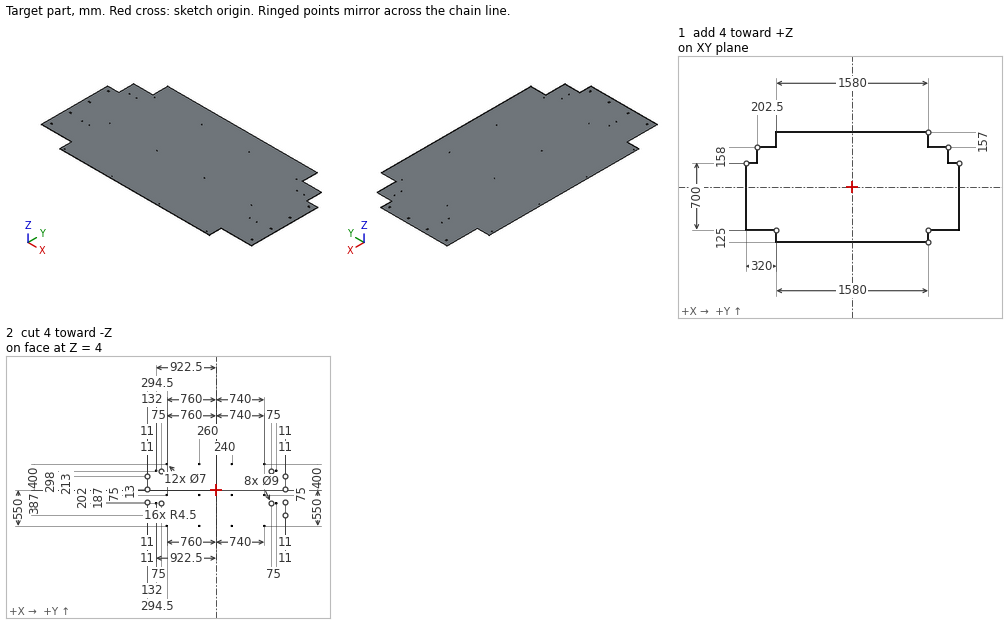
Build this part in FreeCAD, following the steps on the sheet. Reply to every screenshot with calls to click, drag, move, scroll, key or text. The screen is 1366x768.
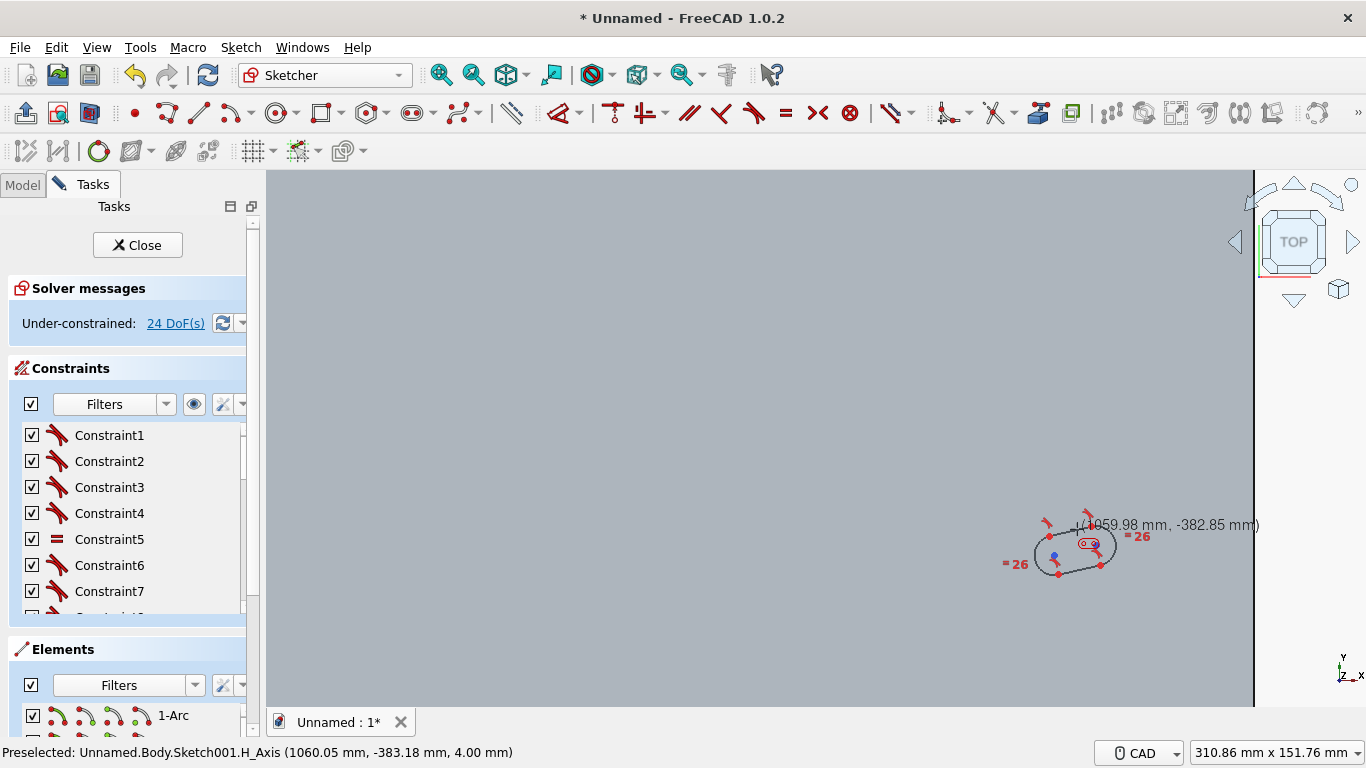
scroll(1089, 538, down, 12)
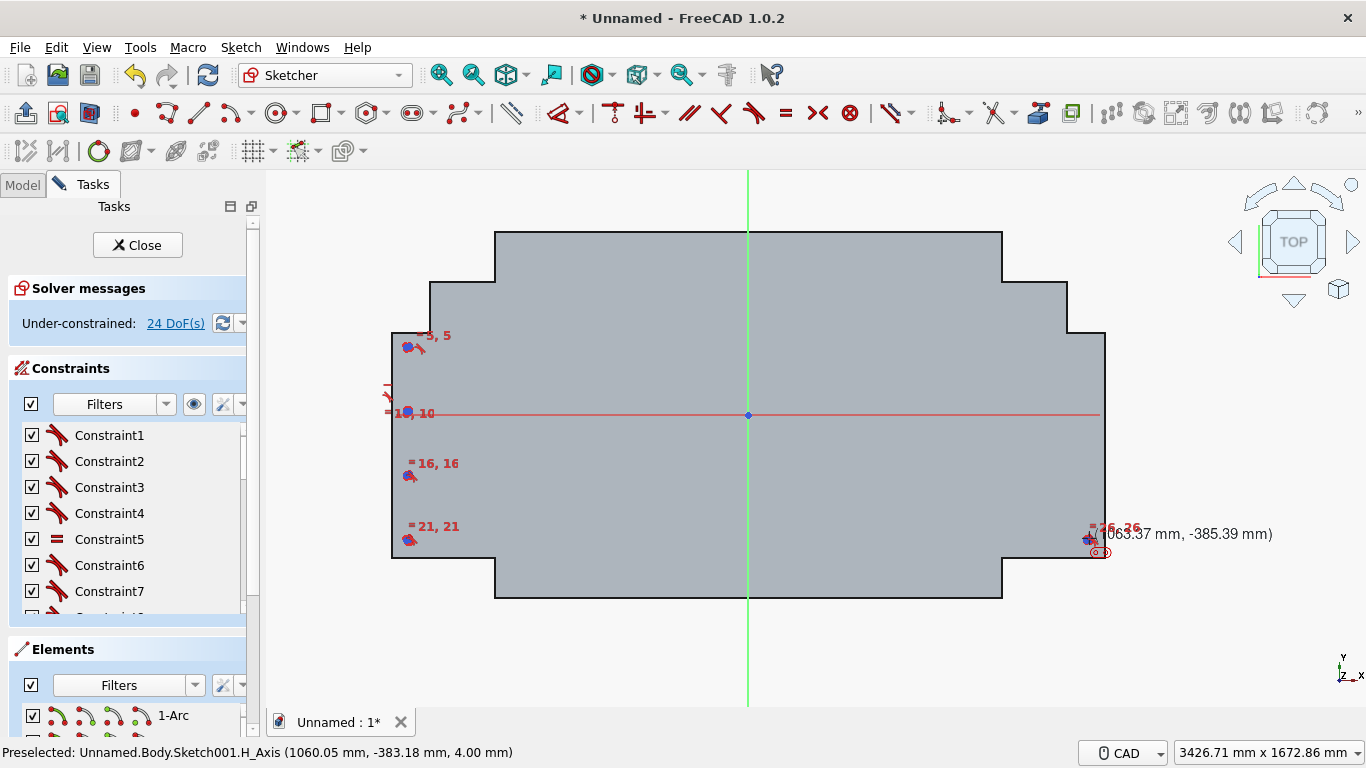
scroll(1087, 475, up, 14)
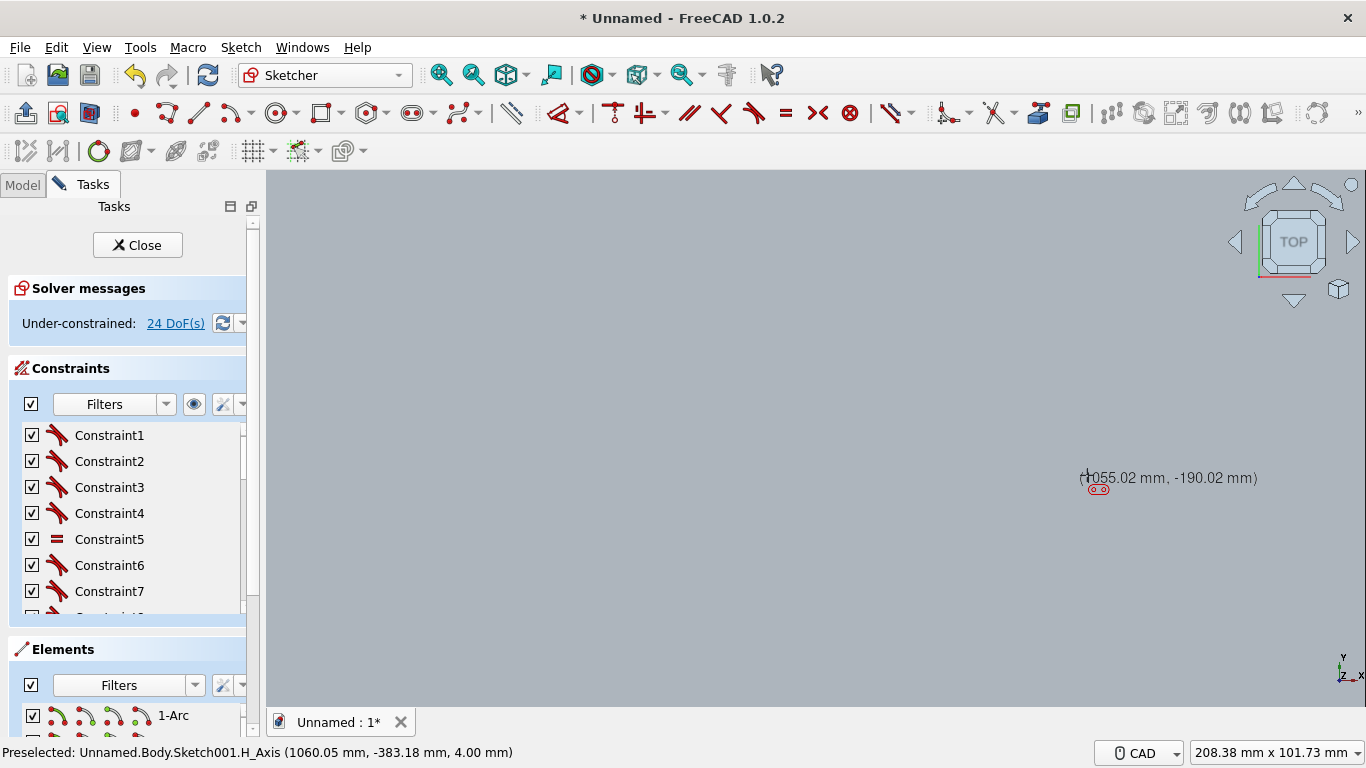
scroll(1087, 475, down, 14)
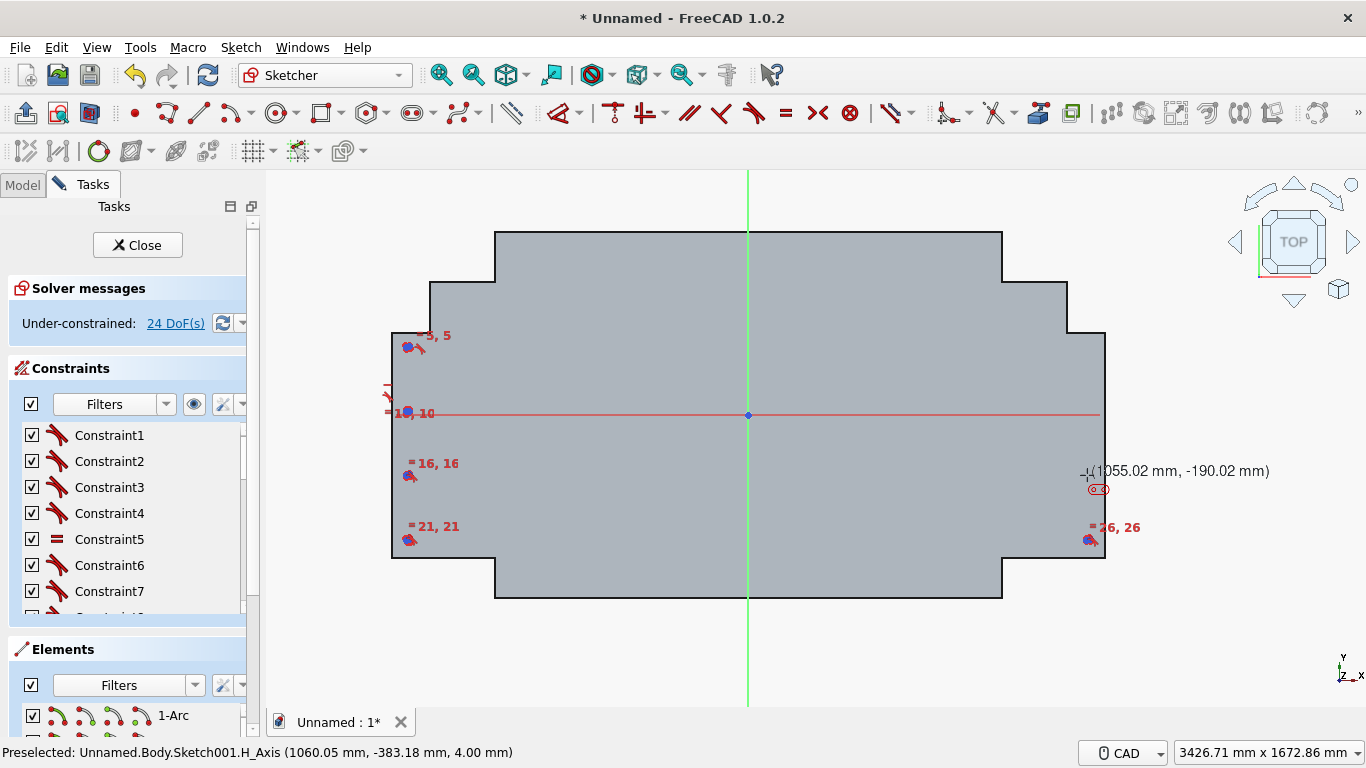
click(1087, 475)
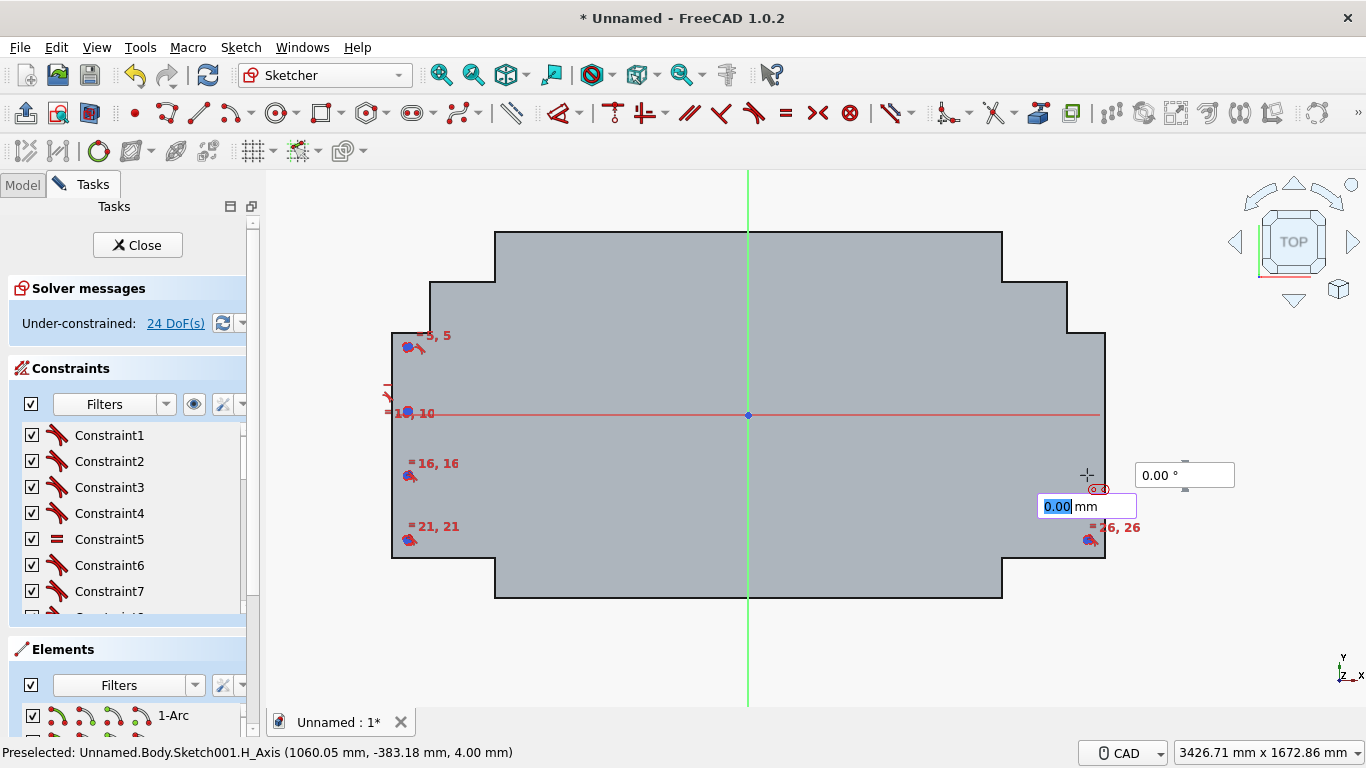
scroll(1090, 475, up, 8)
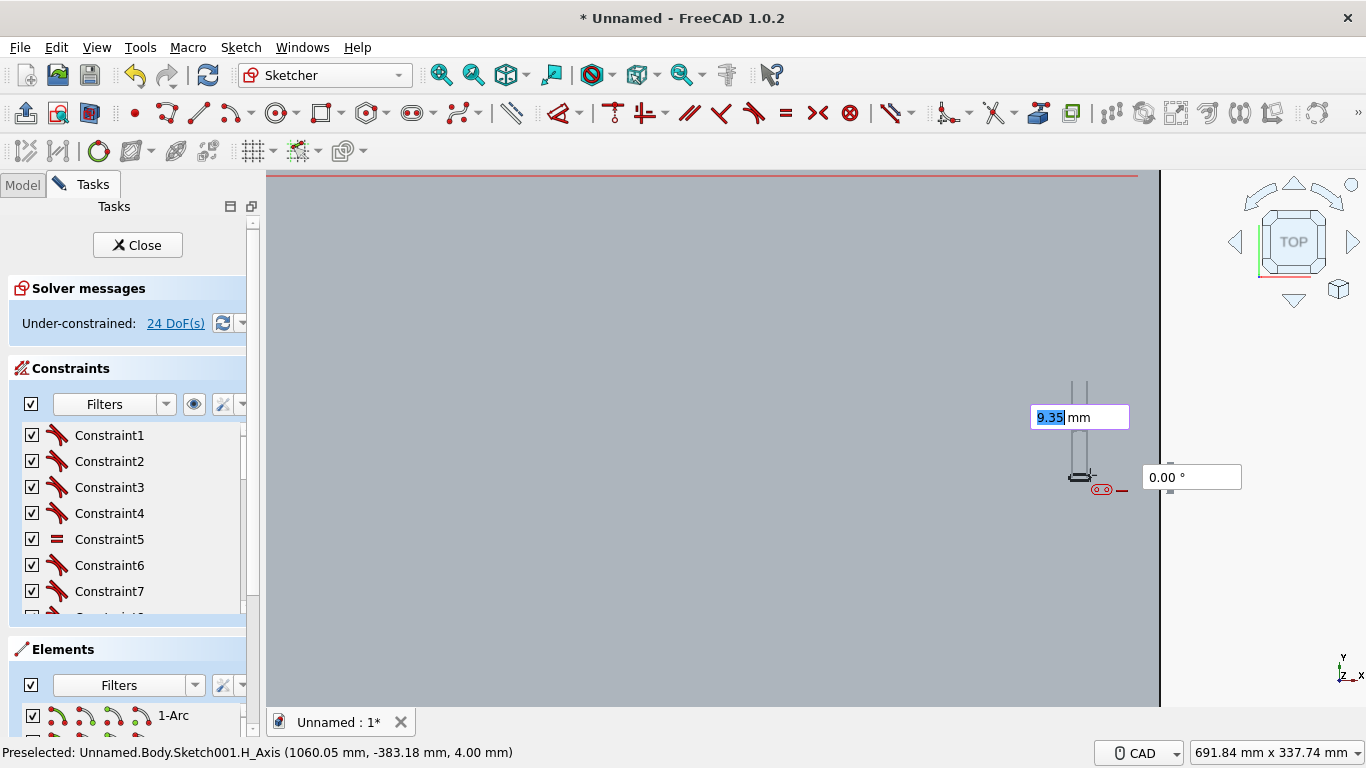
click(1089, 473)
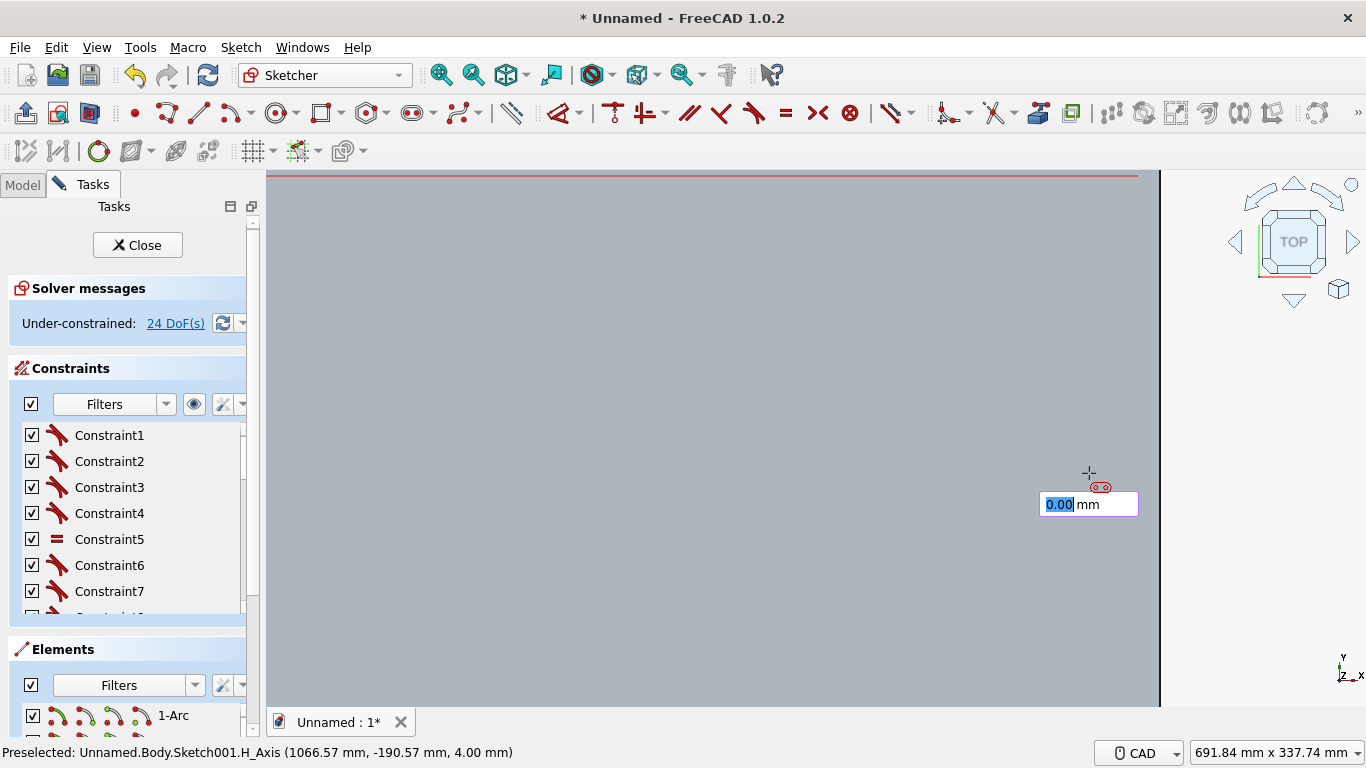
scroll(1080, 466, up, 4)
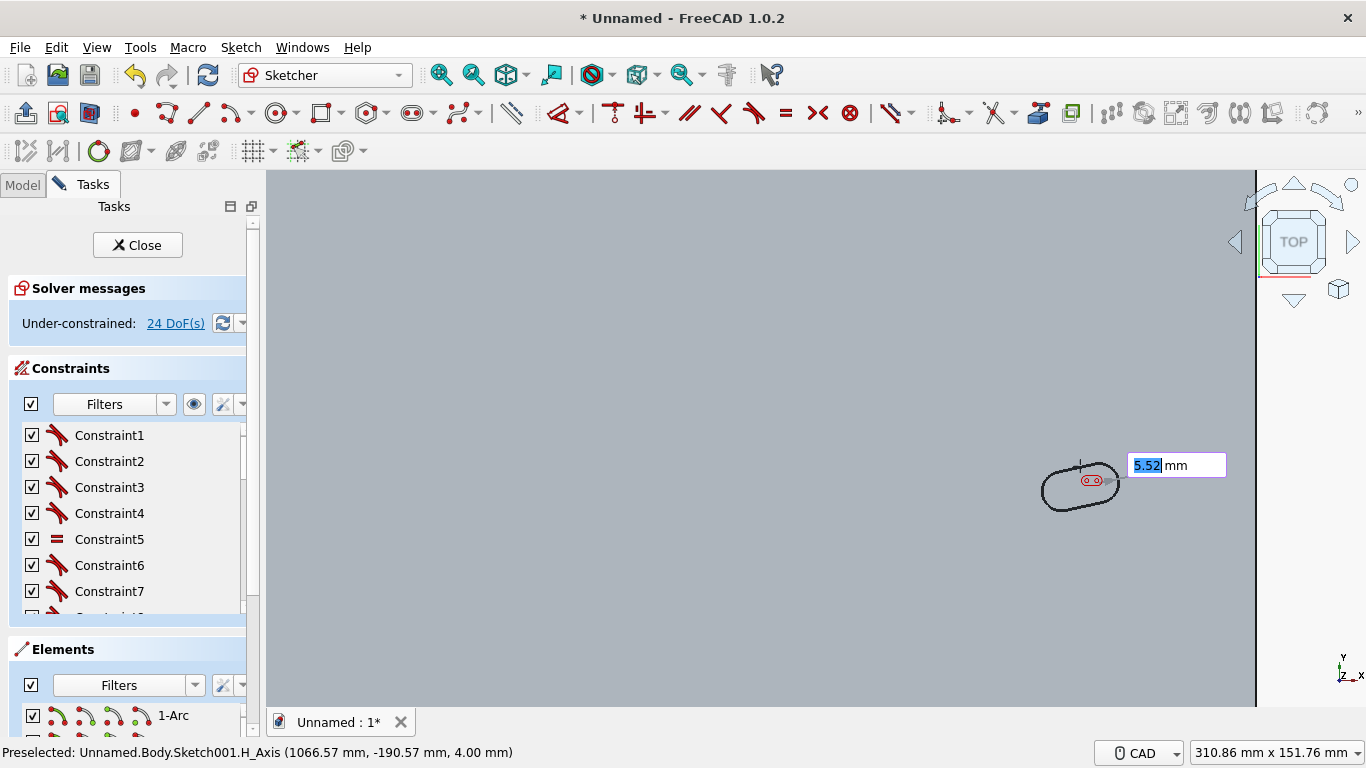
click(1079, 465)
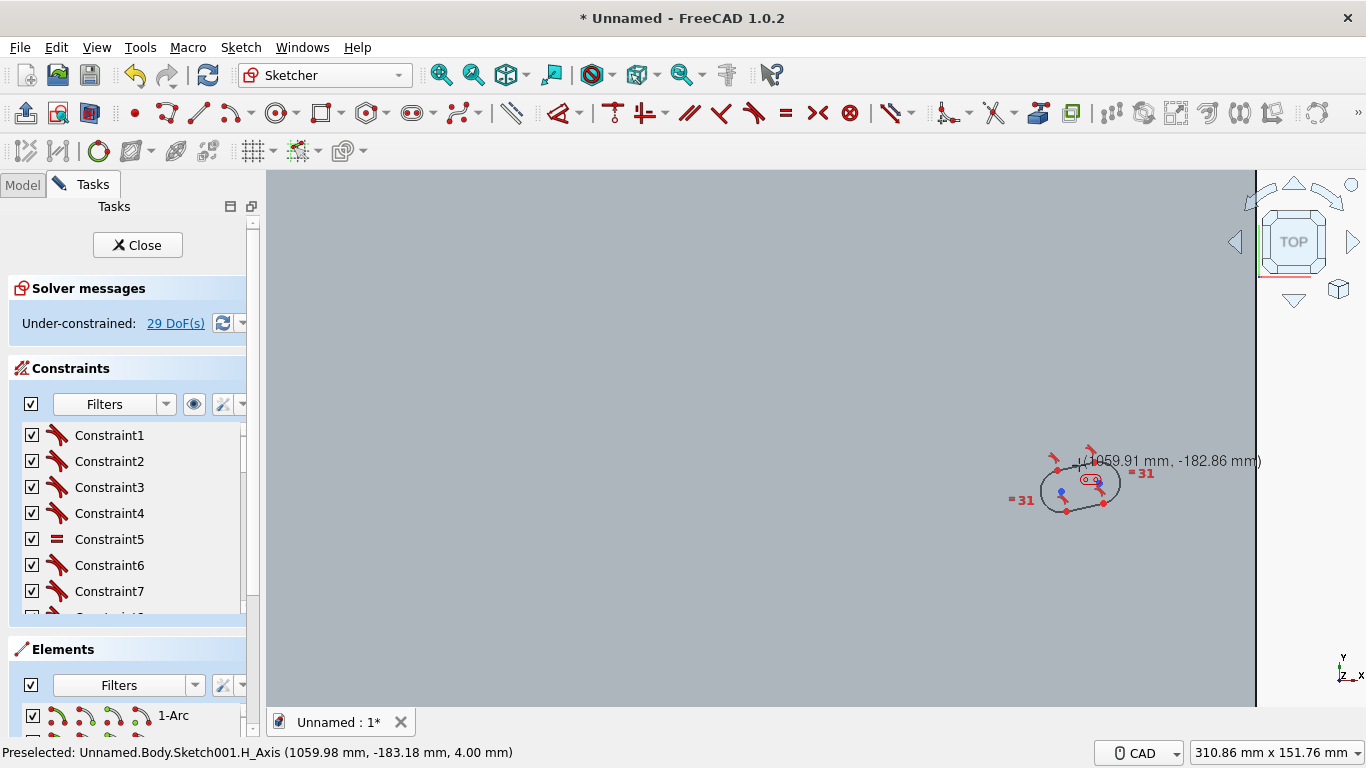
scroll(1089, 474, down, 12)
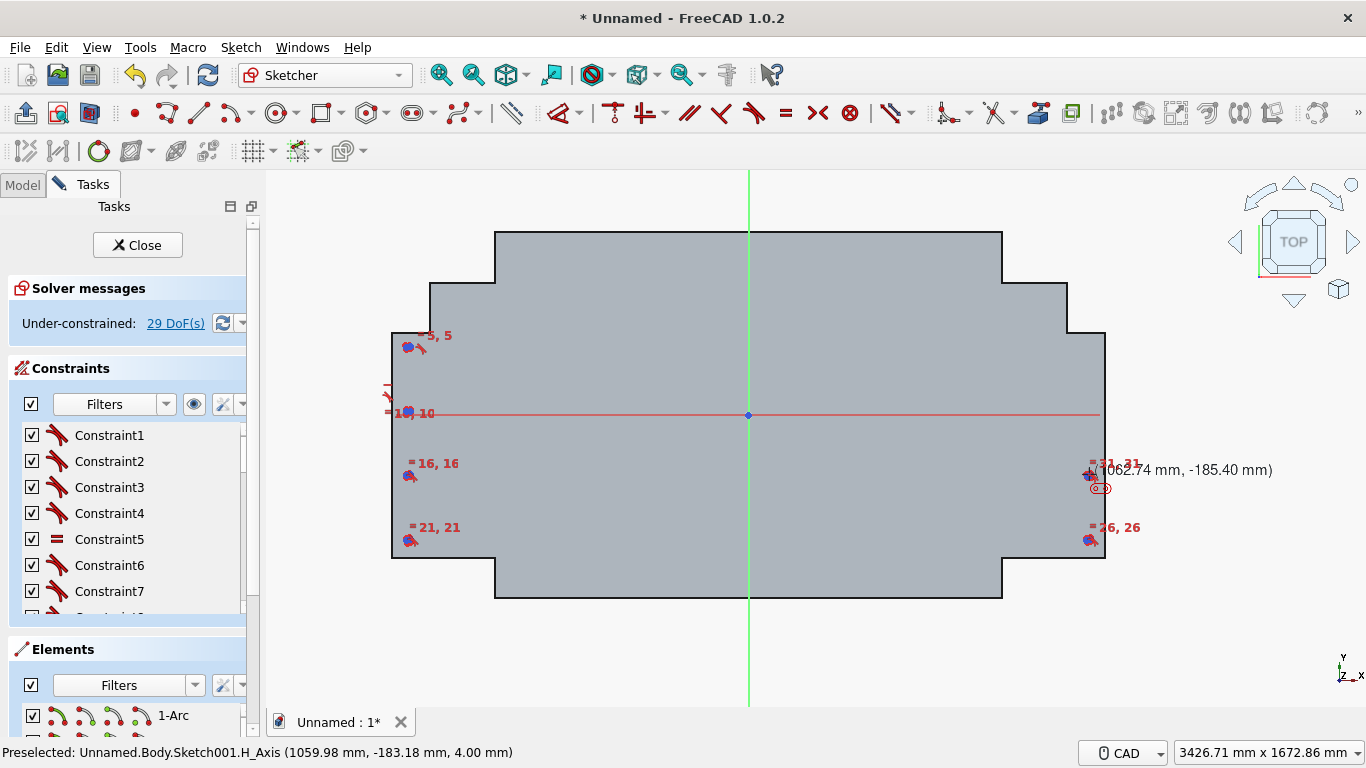
scroll(1087, 411, up, 14)